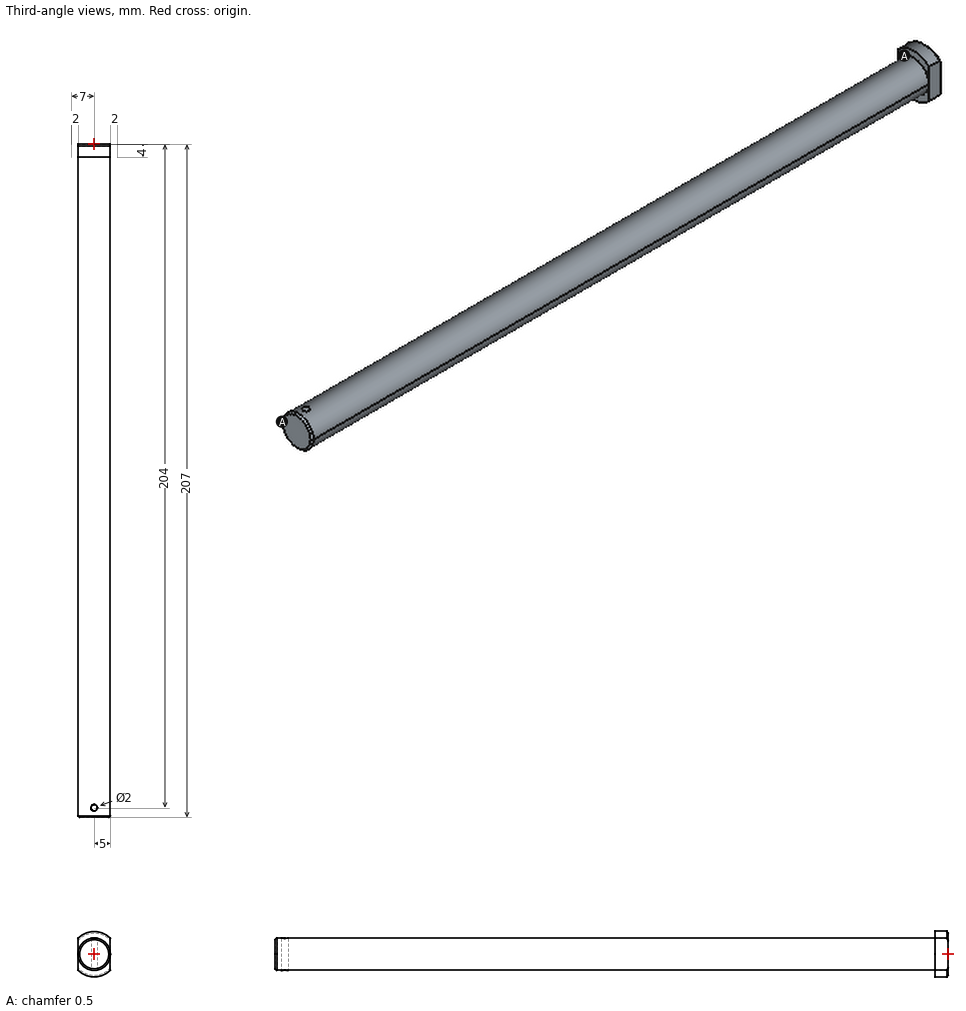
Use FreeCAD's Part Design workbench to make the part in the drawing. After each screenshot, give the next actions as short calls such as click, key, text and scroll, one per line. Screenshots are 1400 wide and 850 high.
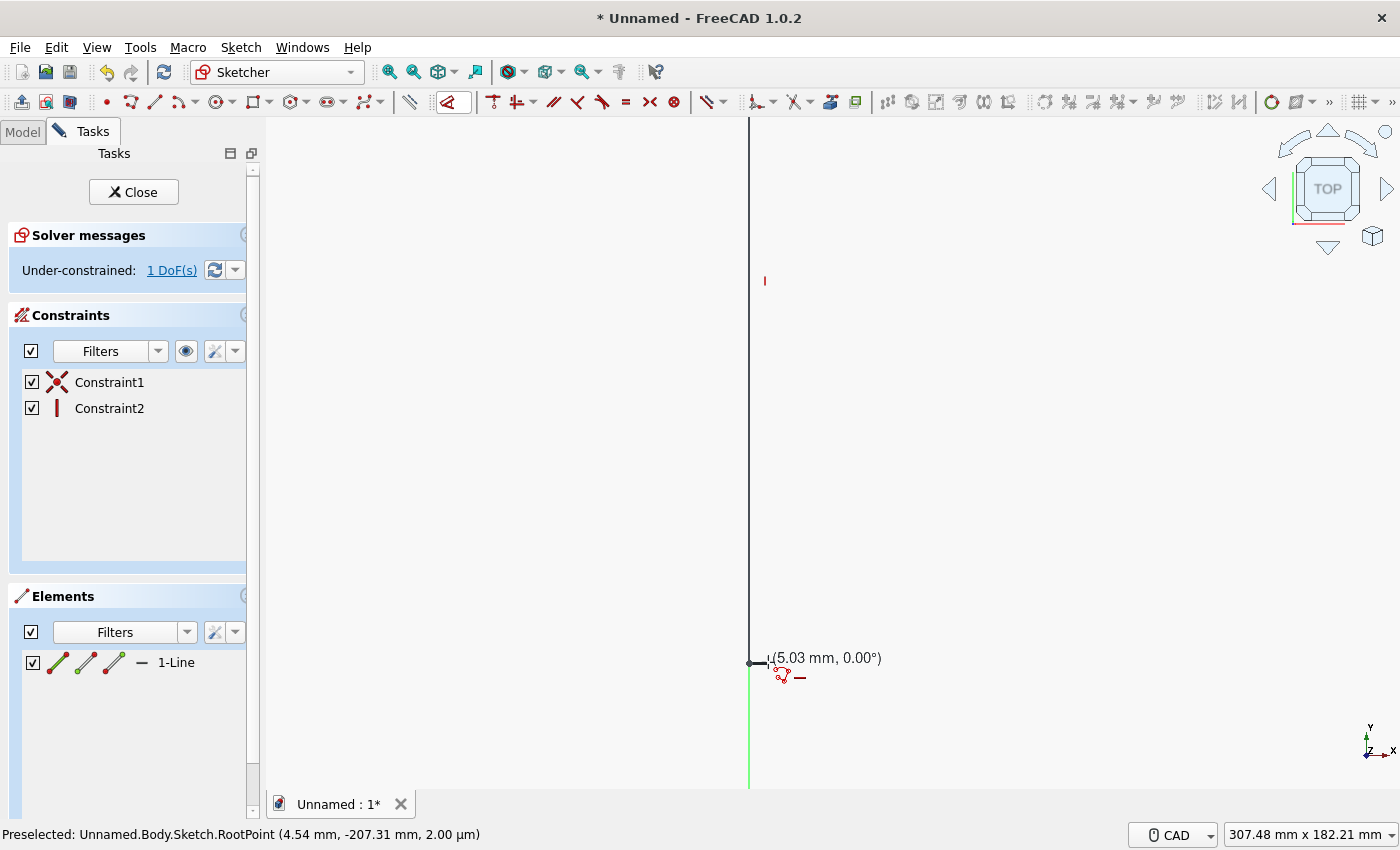
click(768, 661)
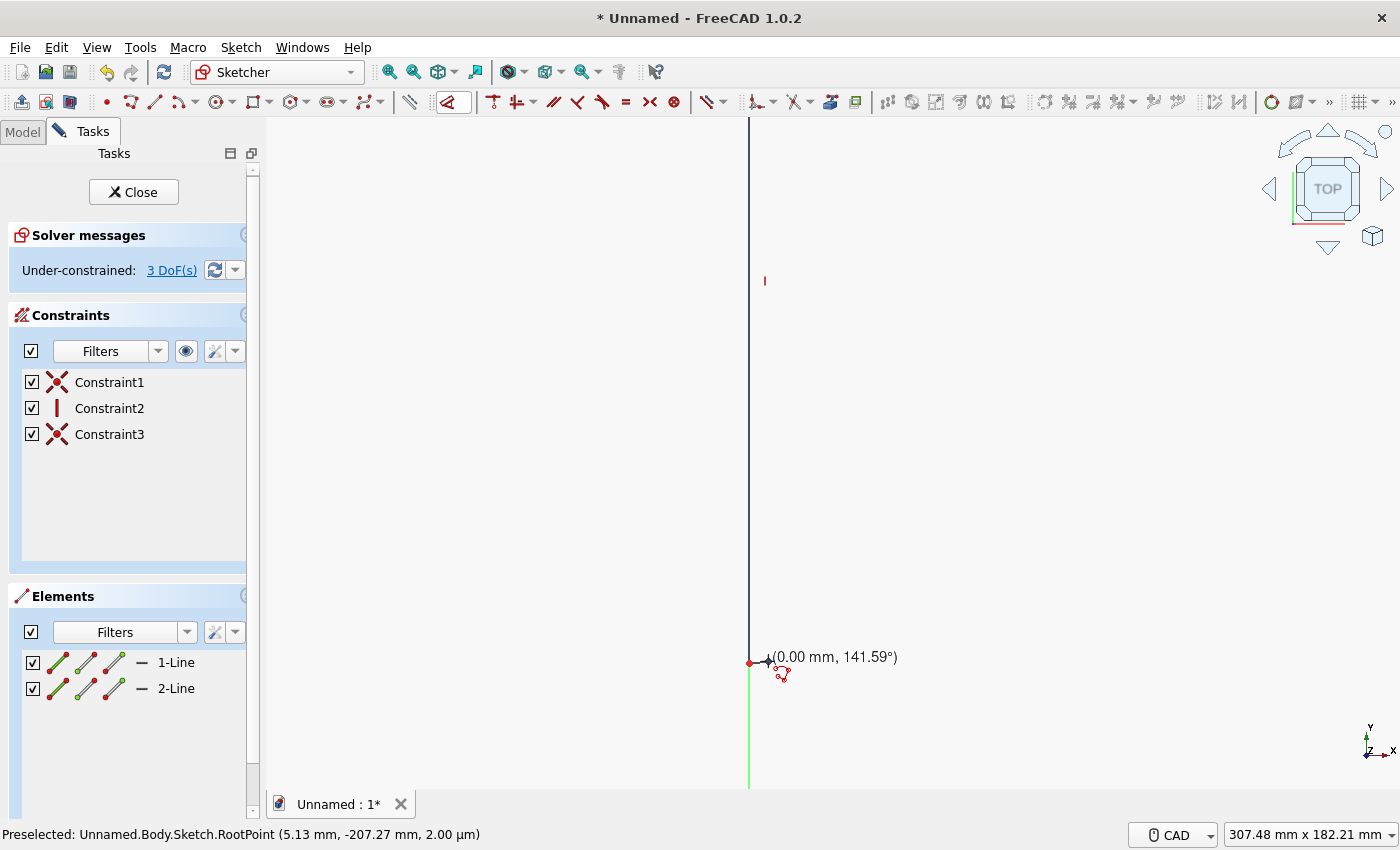
scroll(768, 663, down, 3)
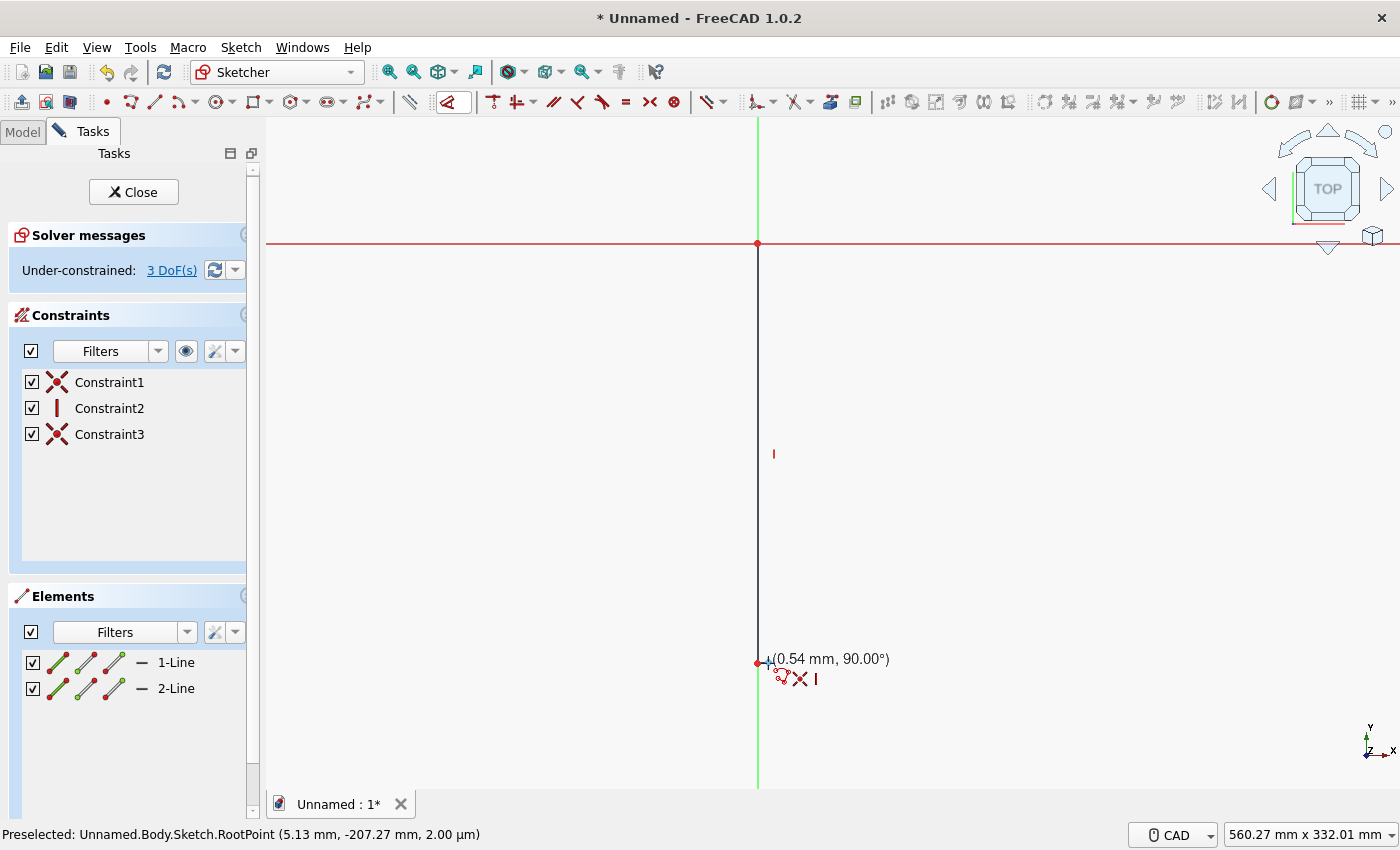
scroll(768, 252, up, 4)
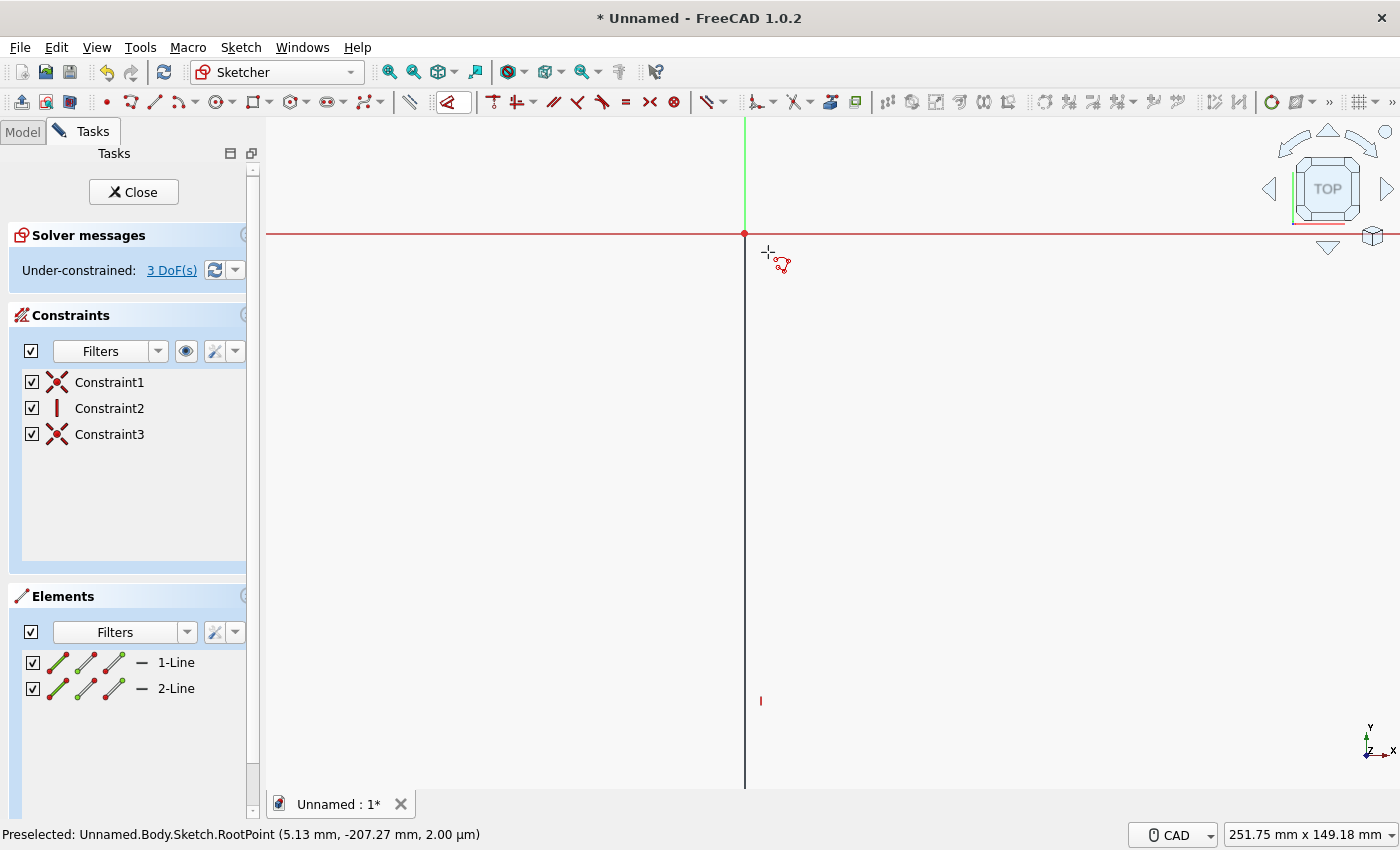
click(768, 252)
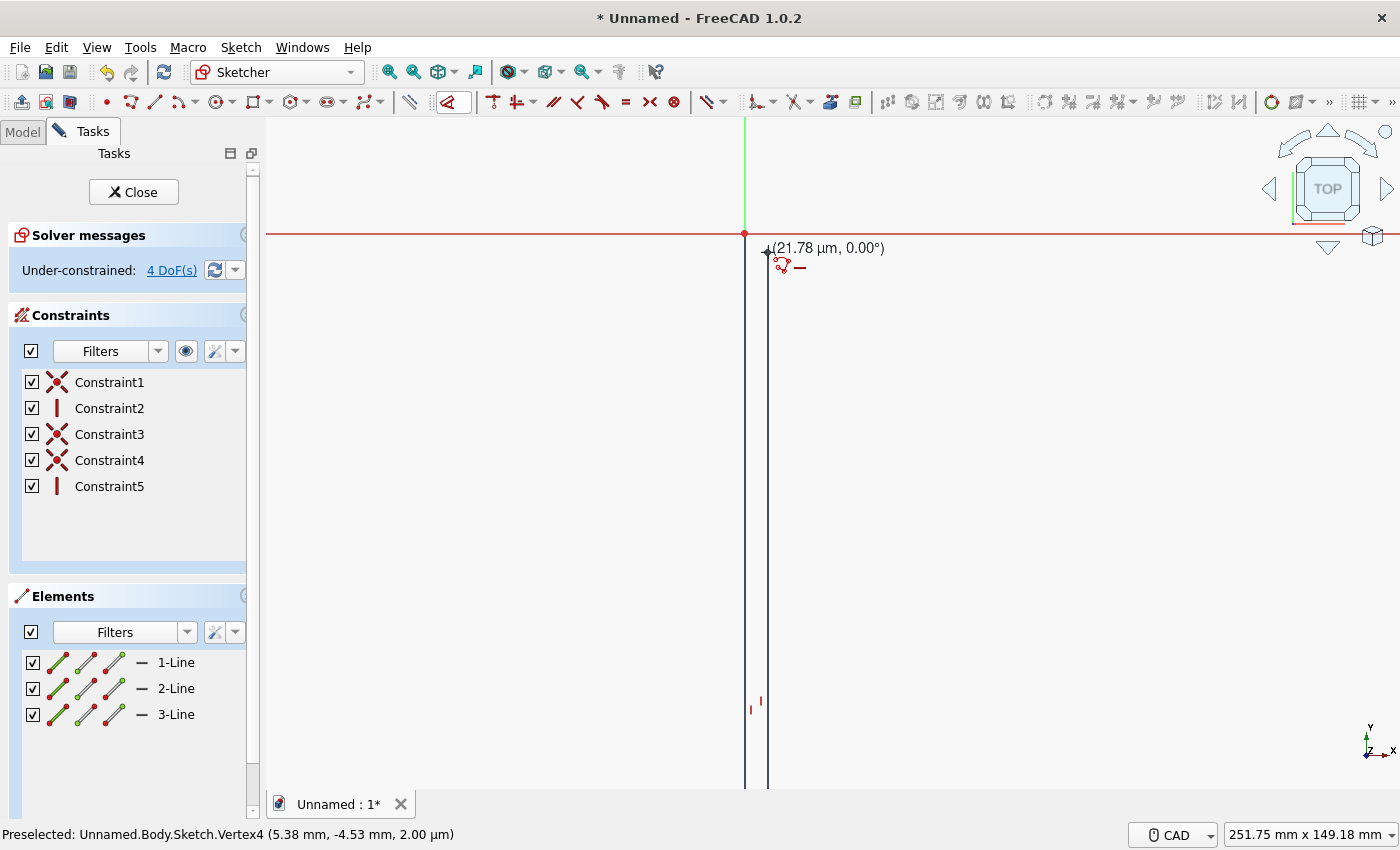
scroll(776, 252, up, 3)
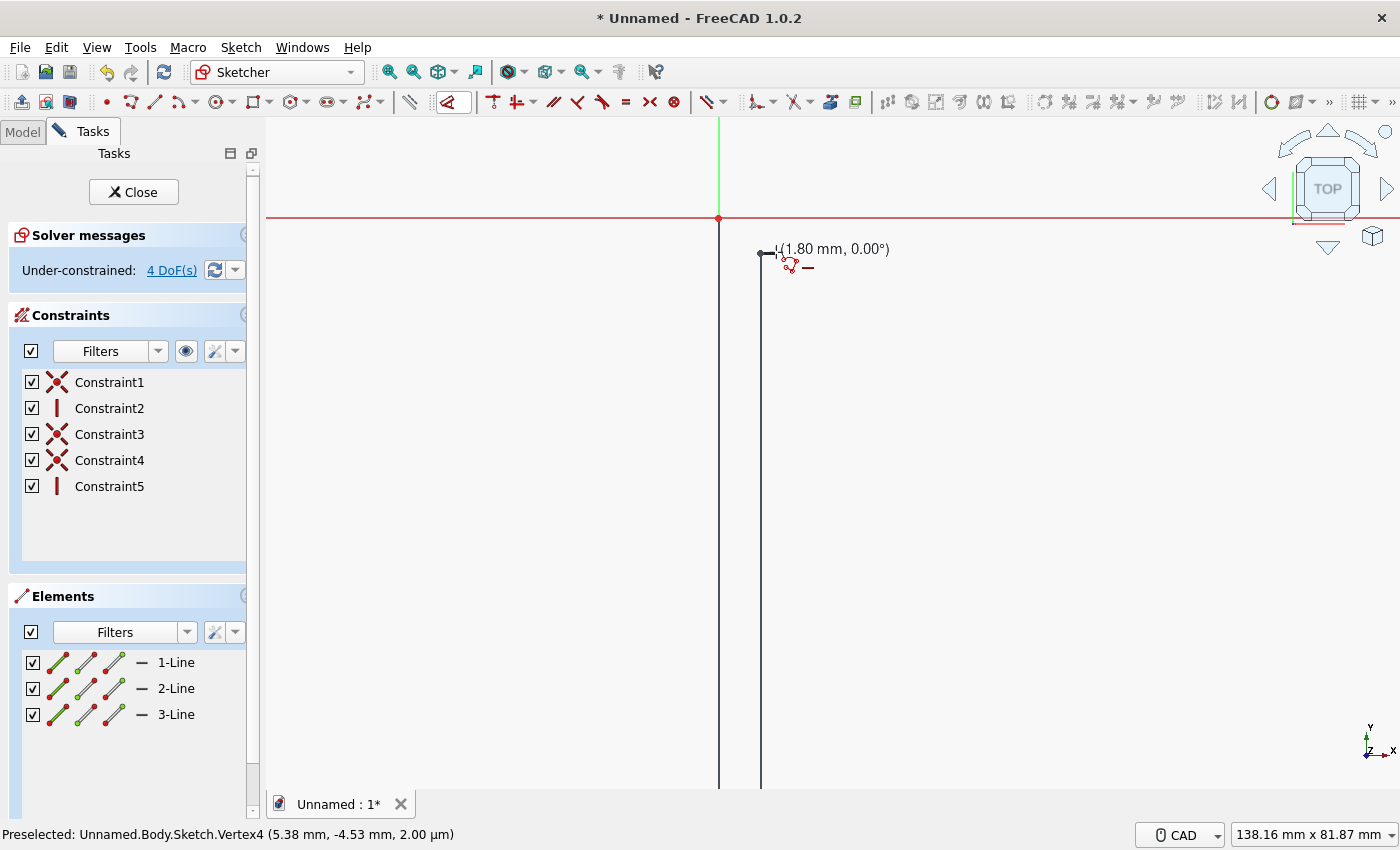
click(776, 252)
click(776, 227)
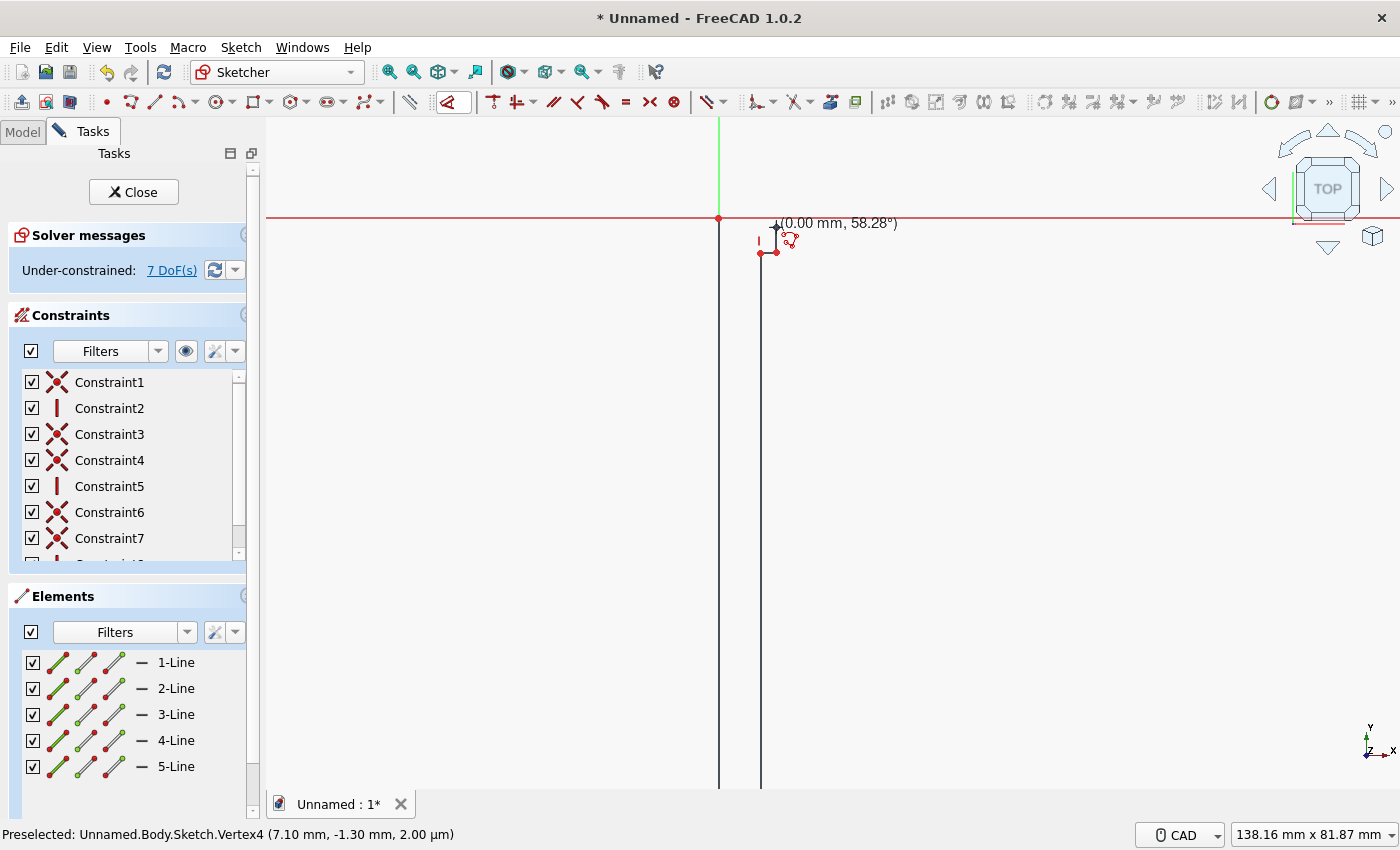
scroll(770, 252, down, 7)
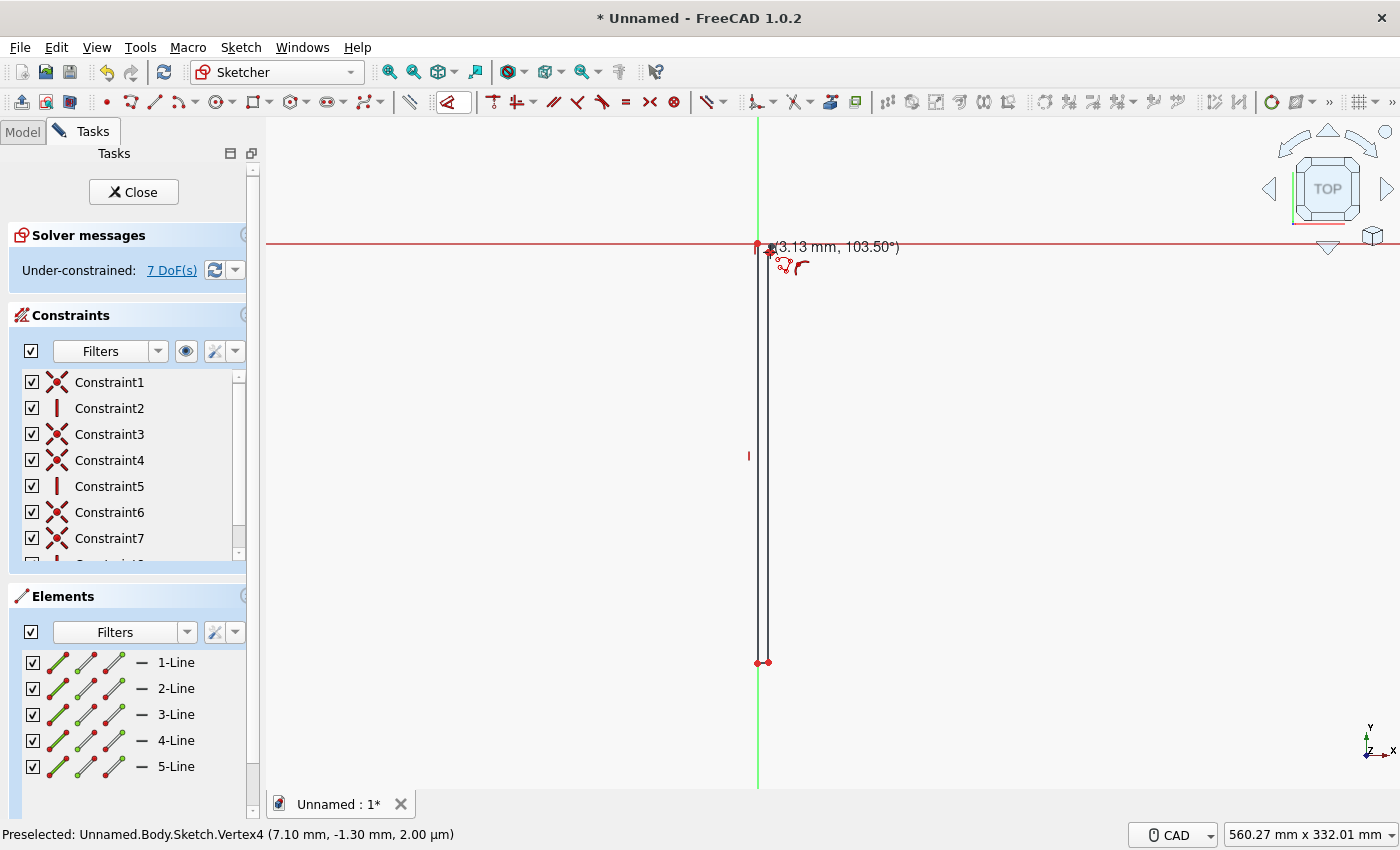
scroll(758, 244, up, 2)